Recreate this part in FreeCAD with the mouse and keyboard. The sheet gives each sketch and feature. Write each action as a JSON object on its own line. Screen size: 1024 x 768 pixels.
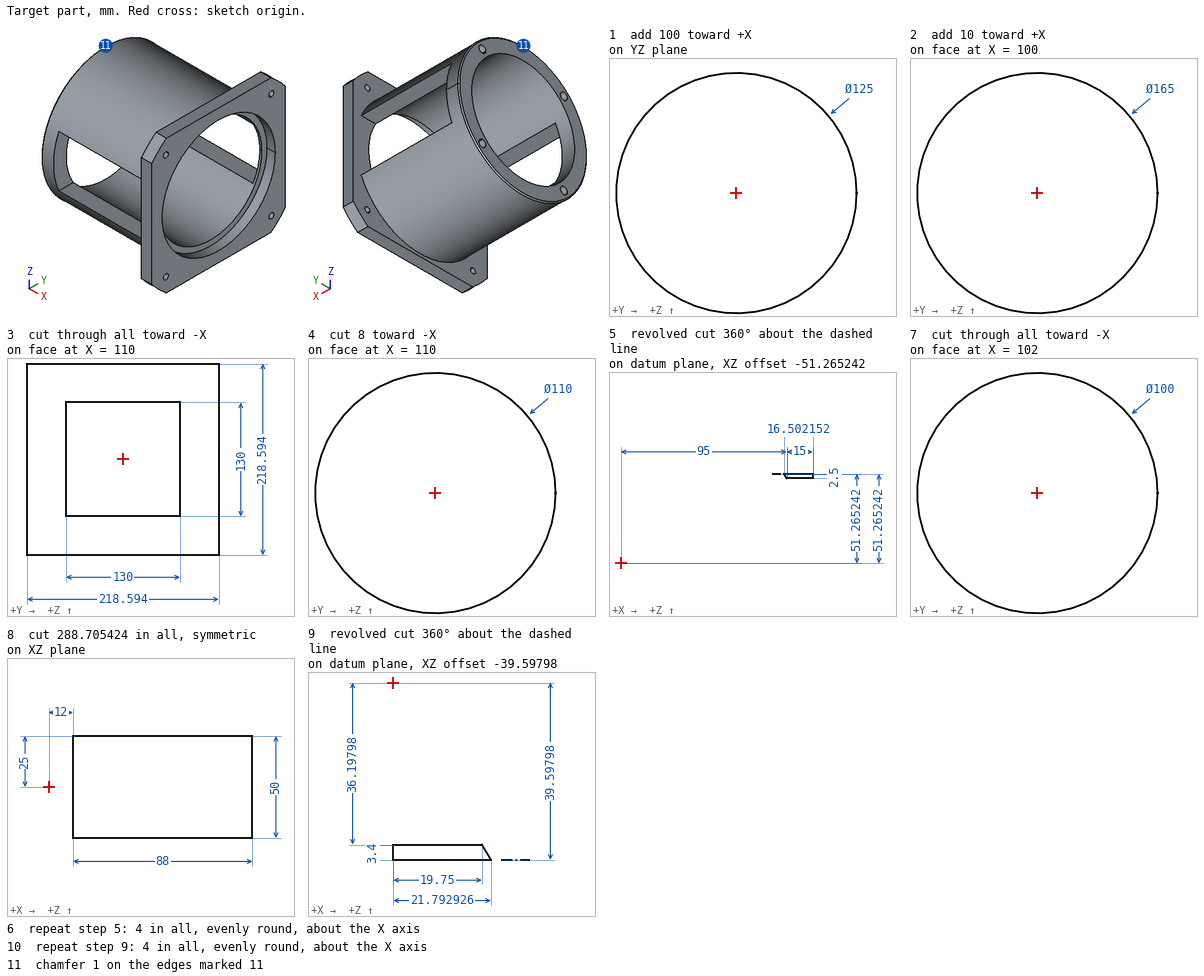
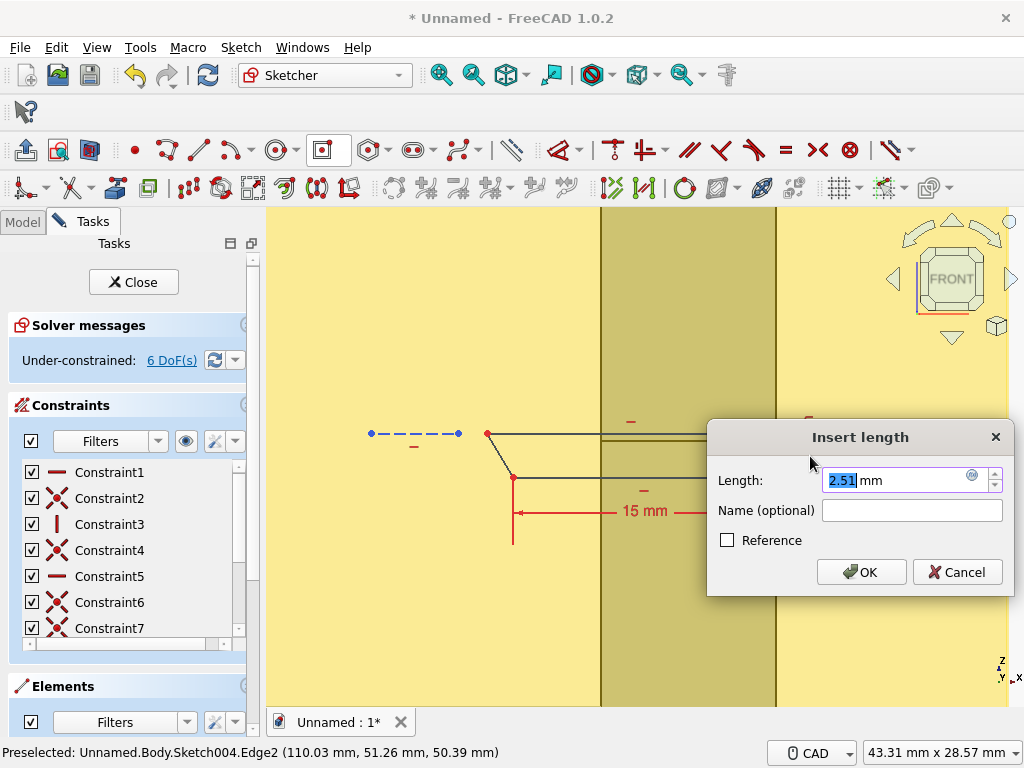
{"action": "type", "text": "2.5"}
{"action": "key", "text": "Return"}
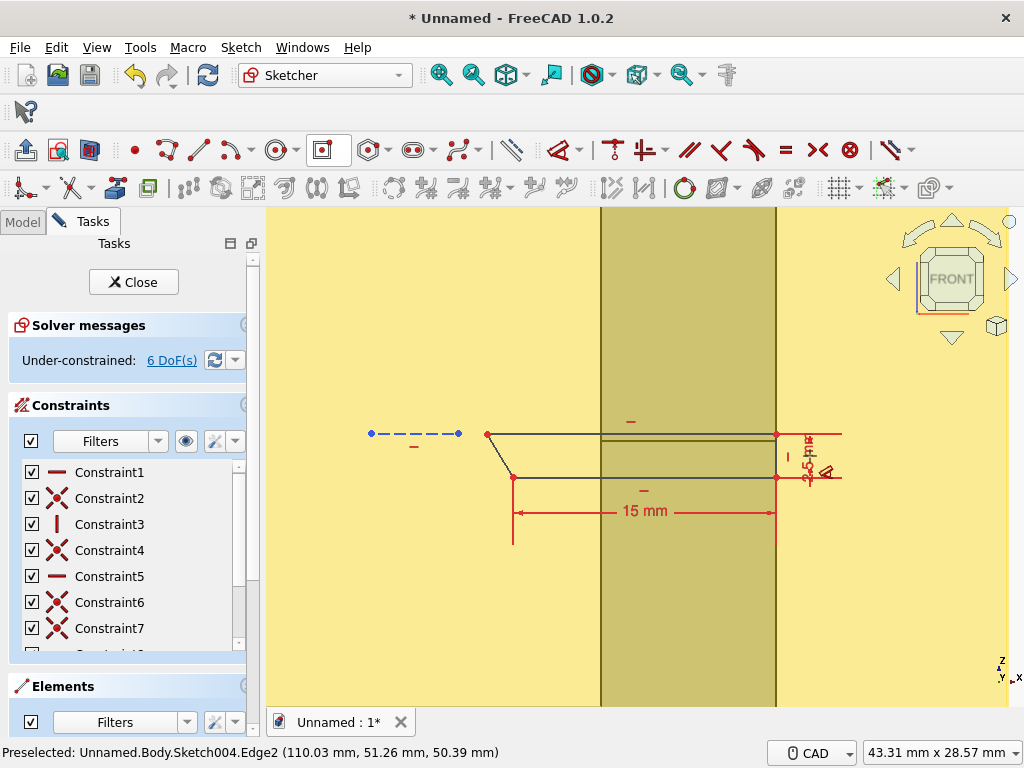
{"action": "left_click", "coordinate": [513, 478]}
{"action": "left_click", "coordinate": [353, 444]}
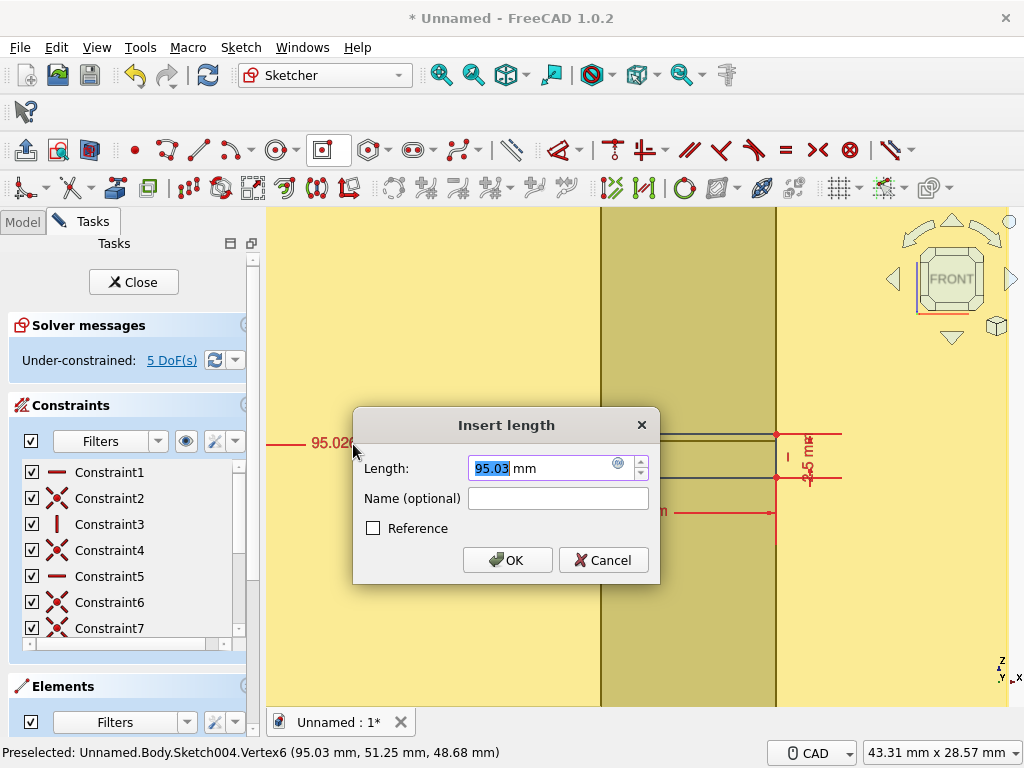
{"action": "type", "text": "95"}
{"action": "key", "text": "Return"}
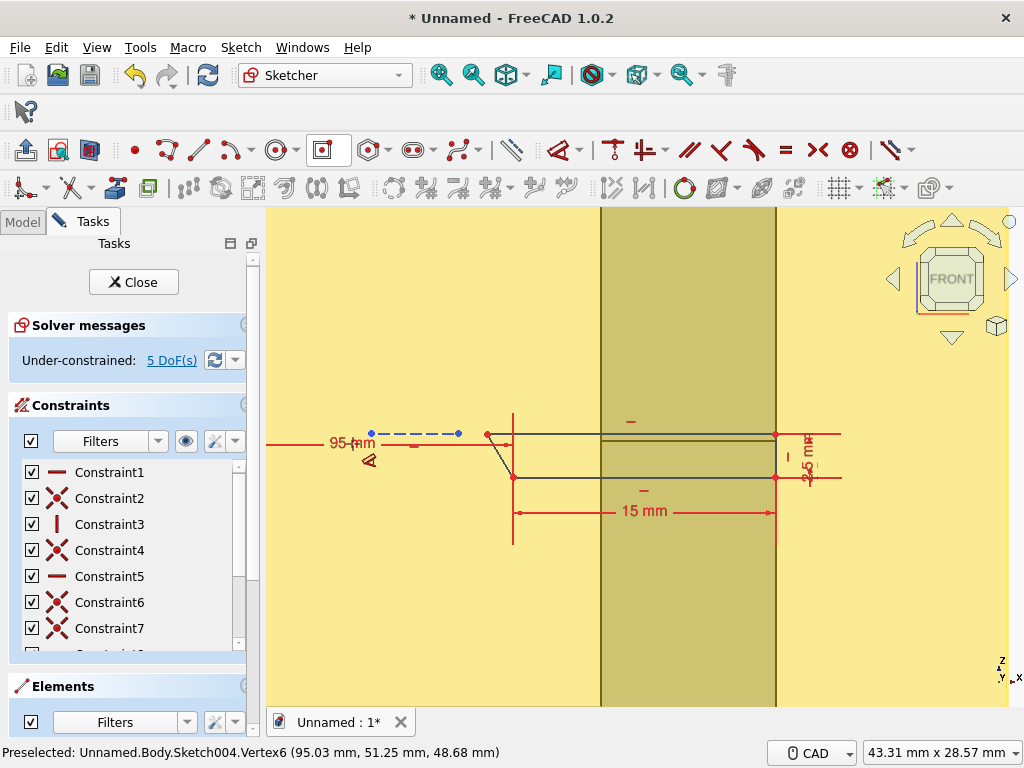
{"action": "left_click", "coordinate": [574, 434]}
{"action": "left_click", "coordinate": [631, 400]}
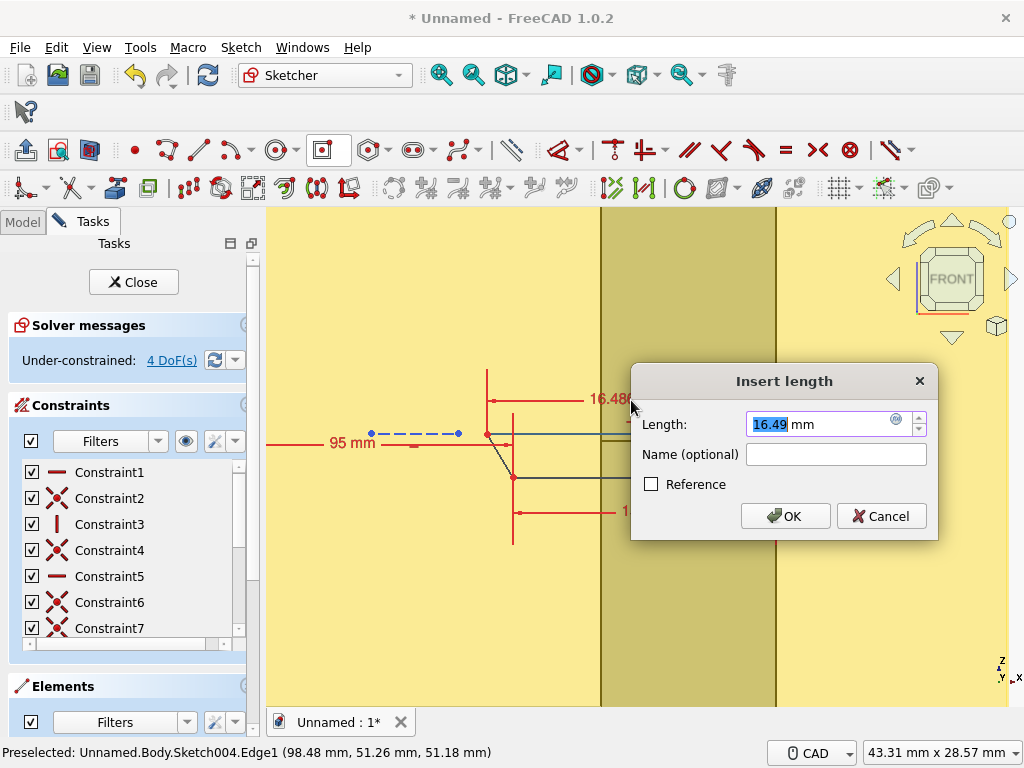
{"action": "type", "text": "16.502152"}
{"action": "key", "text": "Return"}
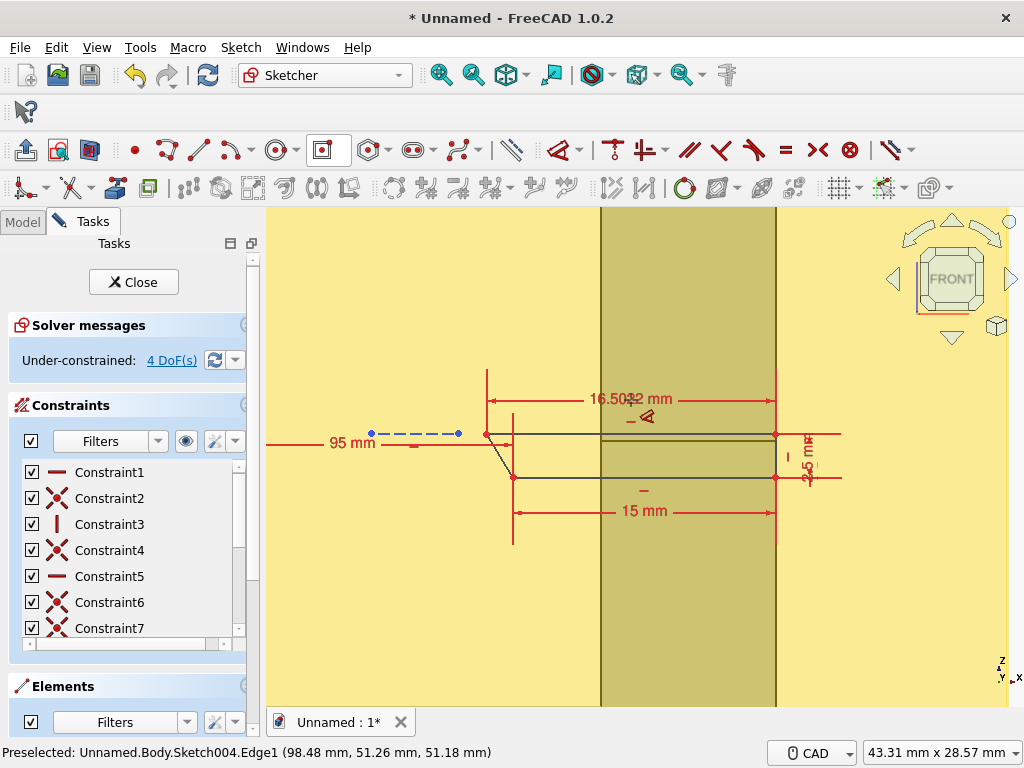
{"action": "left_click", "coordinate": [487, 434]}
{"action": "left_click", "coordinate": [521, 557]}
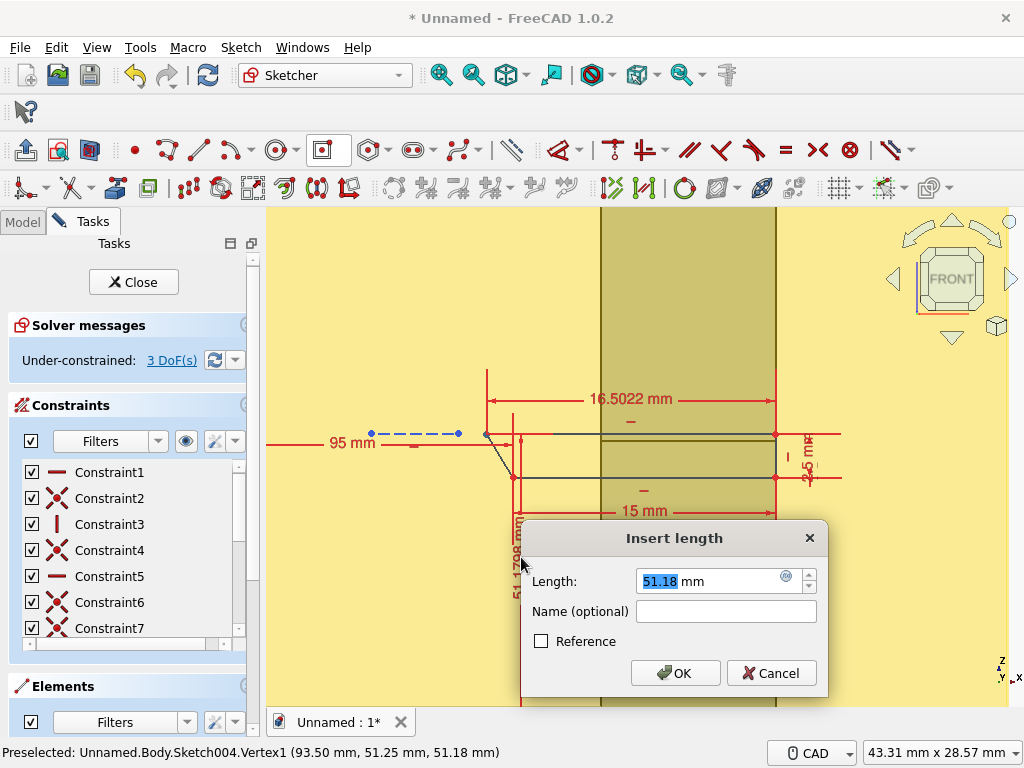
{"action": "type", "text": "51.265242"}
{"action": "key", "text": "Return"}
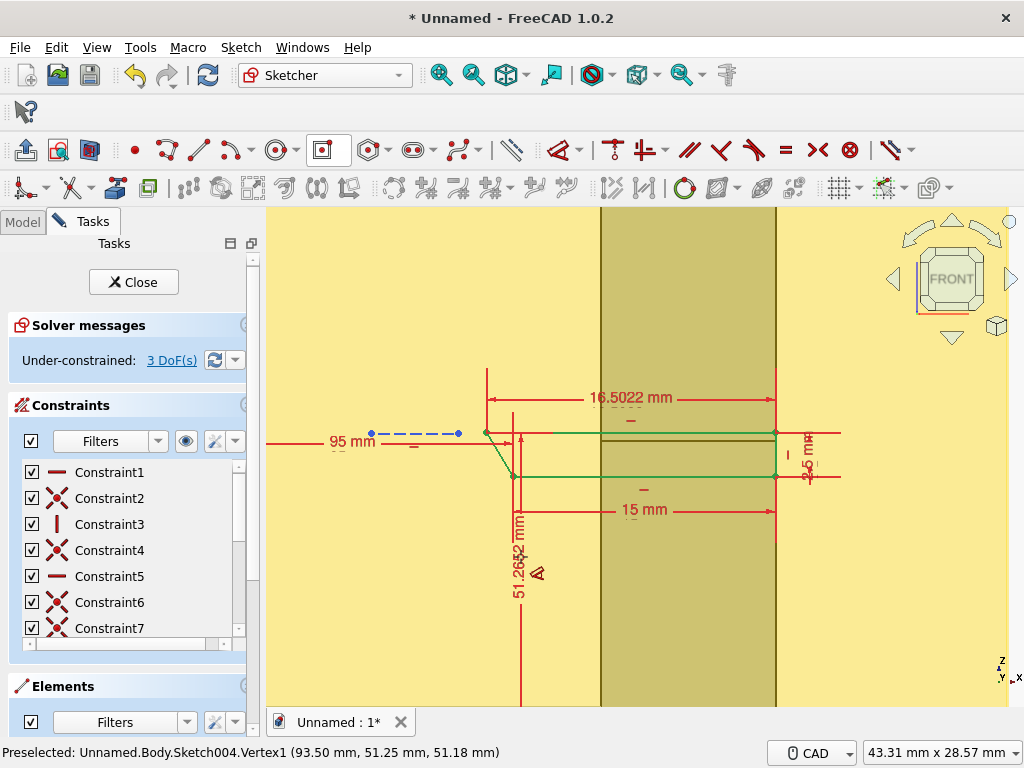
{"action": "left_click", "coordinate": [458, 434]}
{"action": "left_click", "coordinate": [492, 500]}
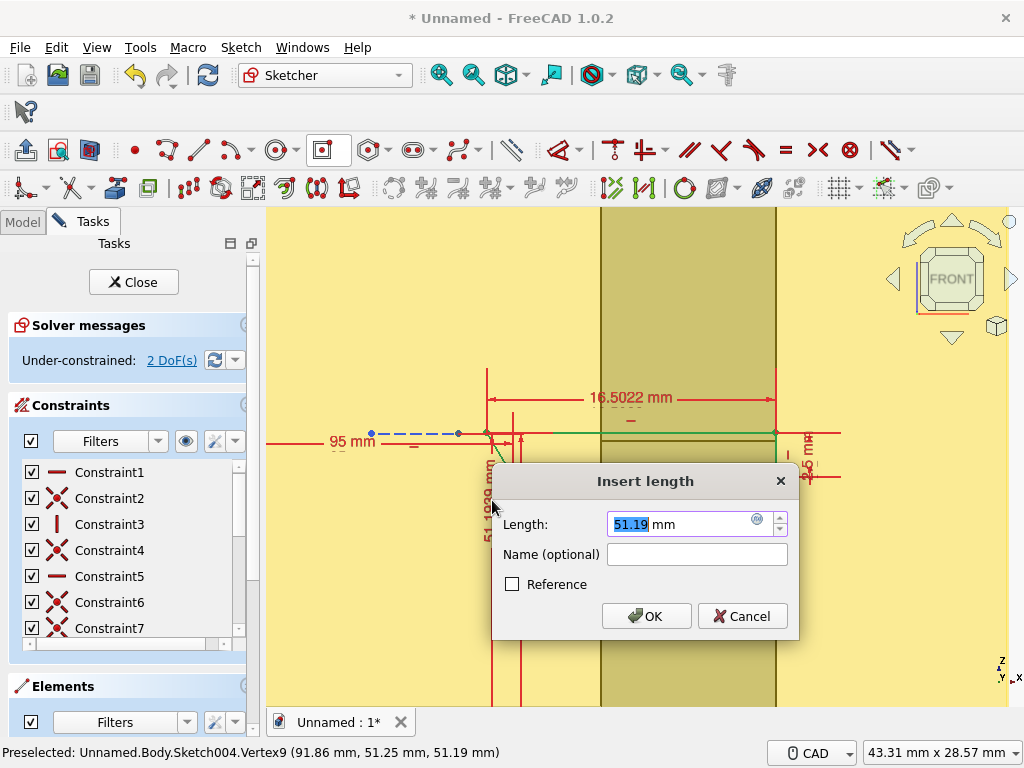
{"action": "type", "text": "51.265242"}
{"action": "key", "text": "Return"}
{"action": "key", "text": "Escape"}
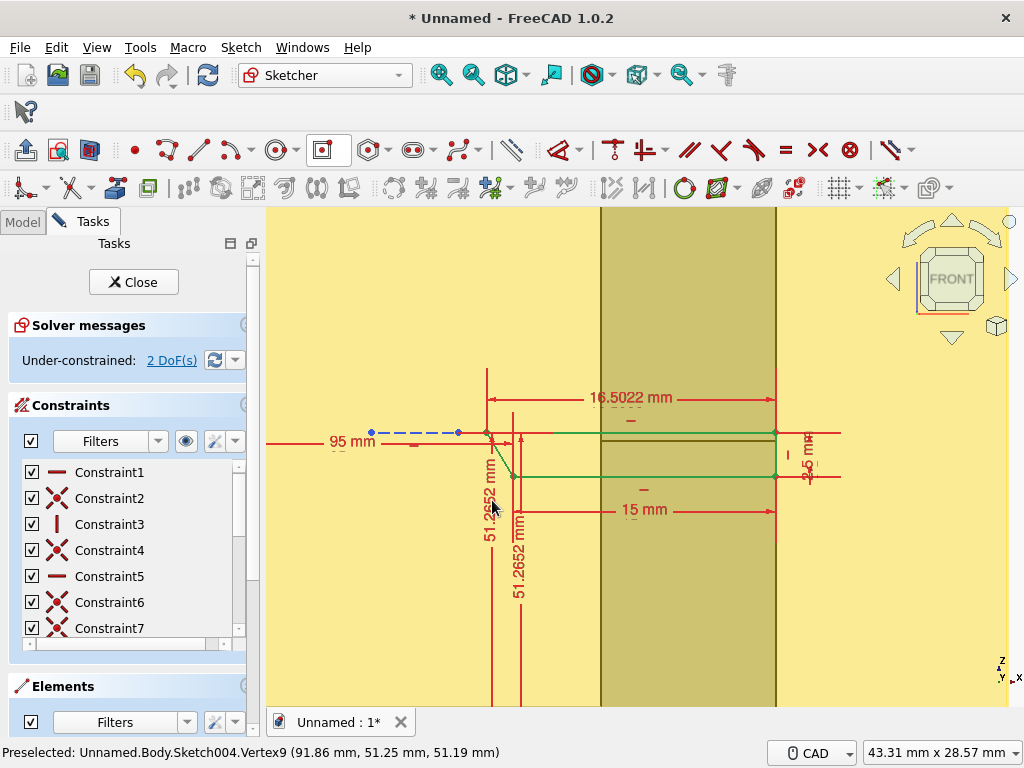
{"action": "left_click", "coordinate": [134, 282]}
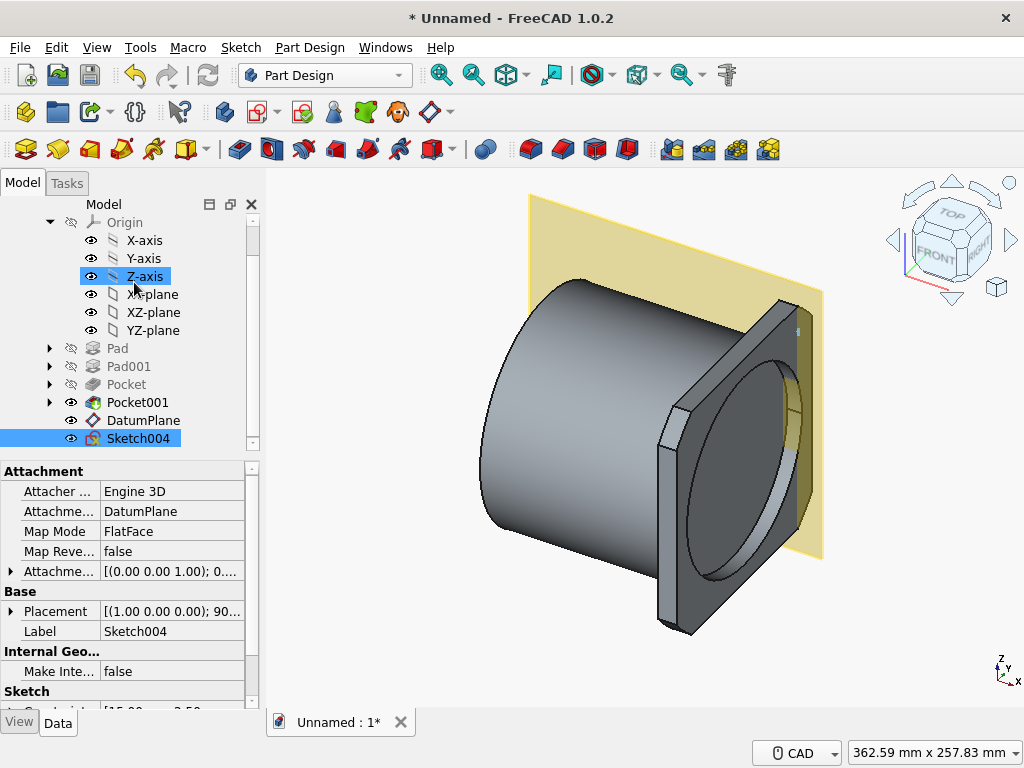
{"action": "left_click", "coordinate": [304, 150]}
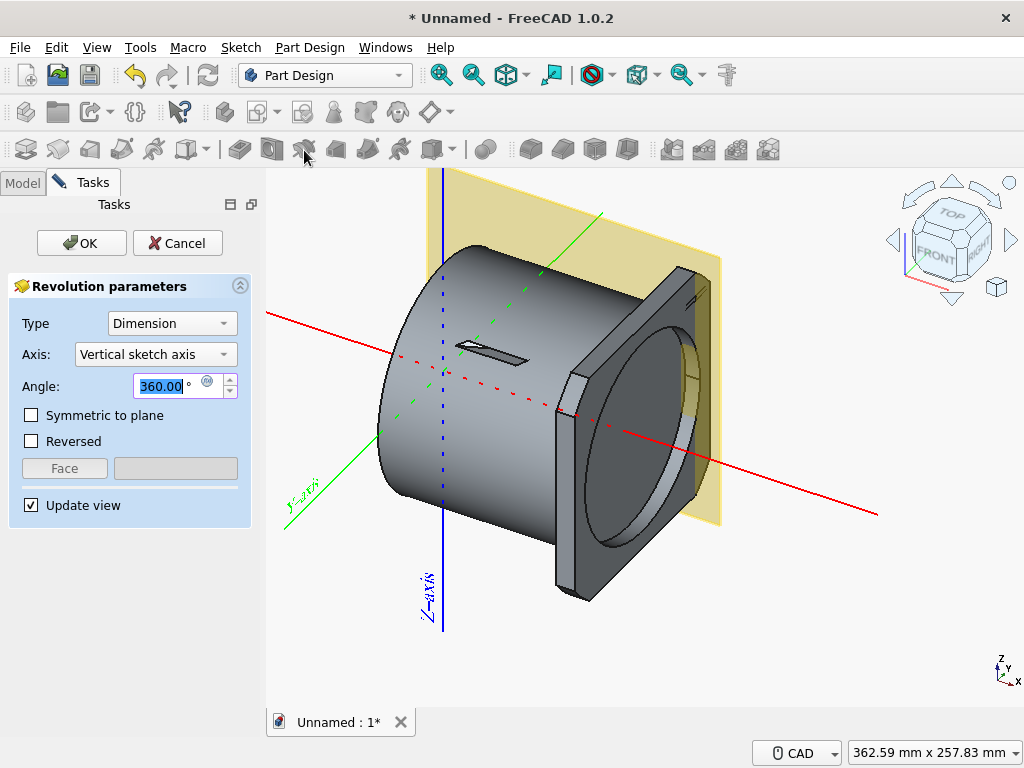
{"action": "left_click", "coordinate": [156, 354]}